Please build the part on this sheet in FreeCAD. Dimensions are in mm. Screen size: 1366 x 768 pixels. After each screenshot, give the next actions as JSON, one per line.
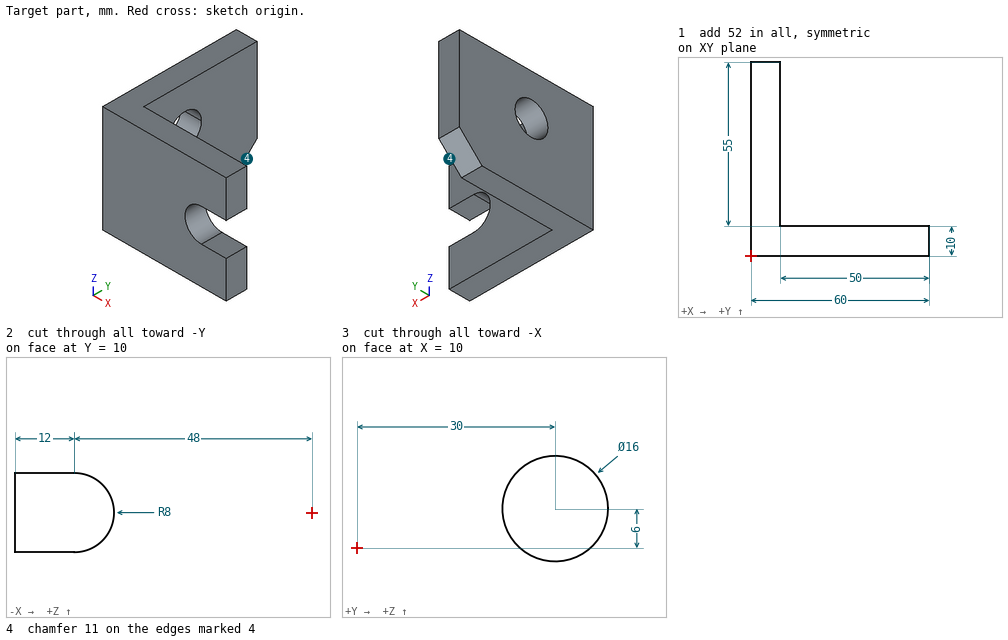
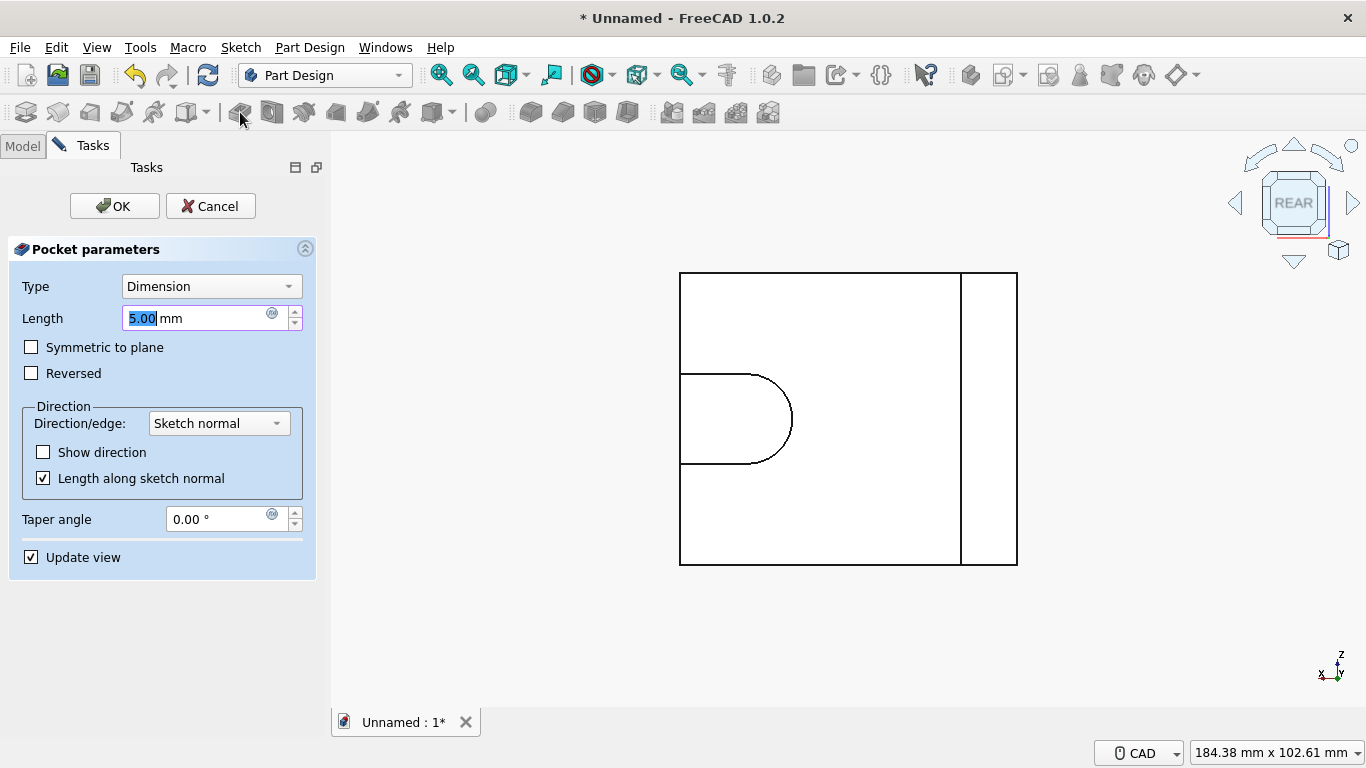
{"action": "left_click", "coordinate": [212, 286]}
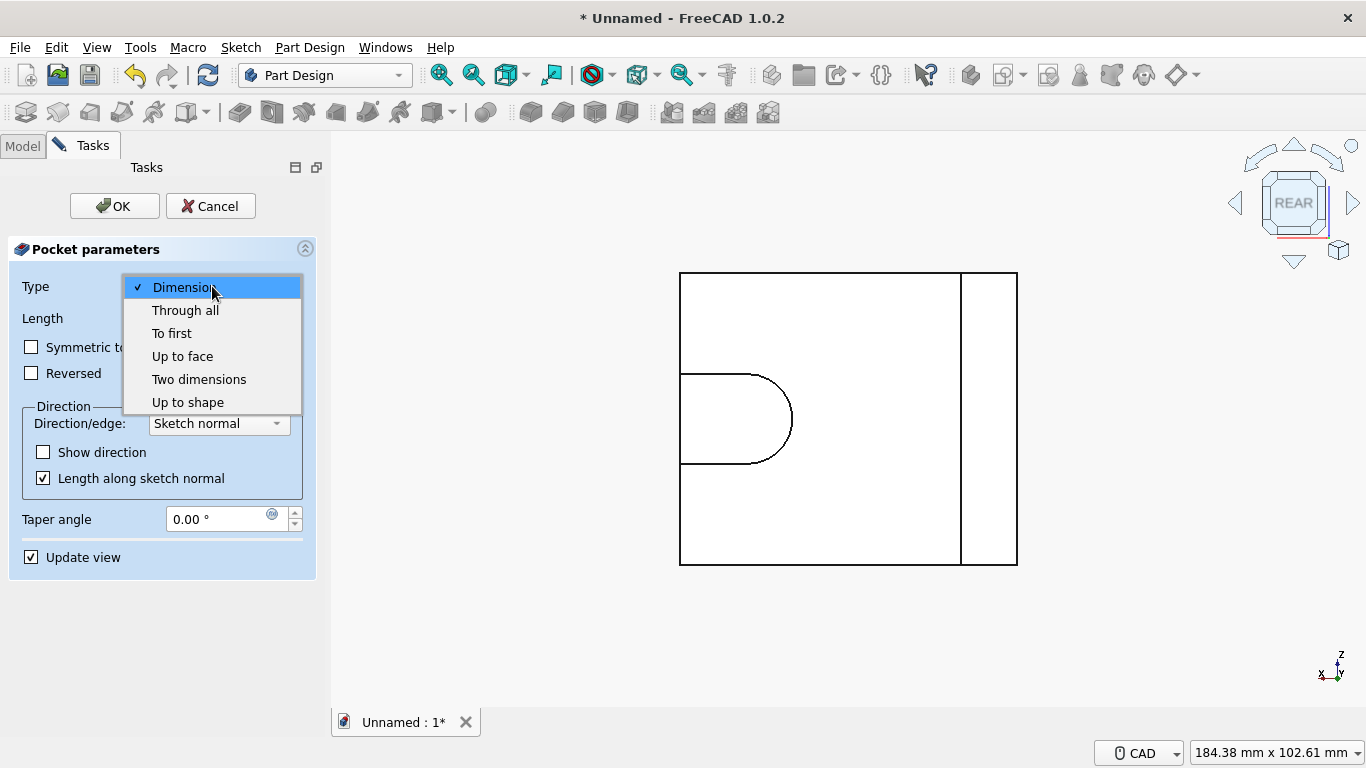
{"action": "left_click", "coordinate": [212, 310]}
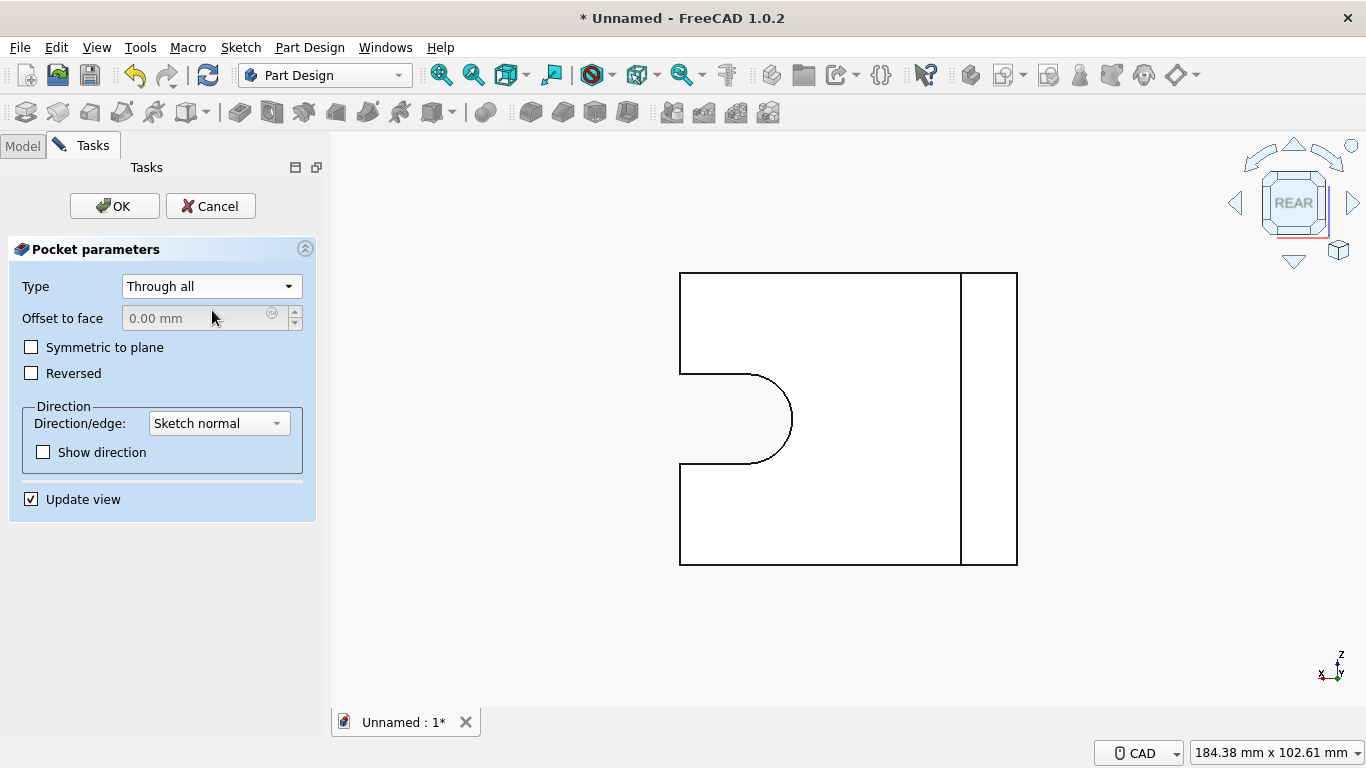
{"action": "left_click", "coordinate": [115, 206]}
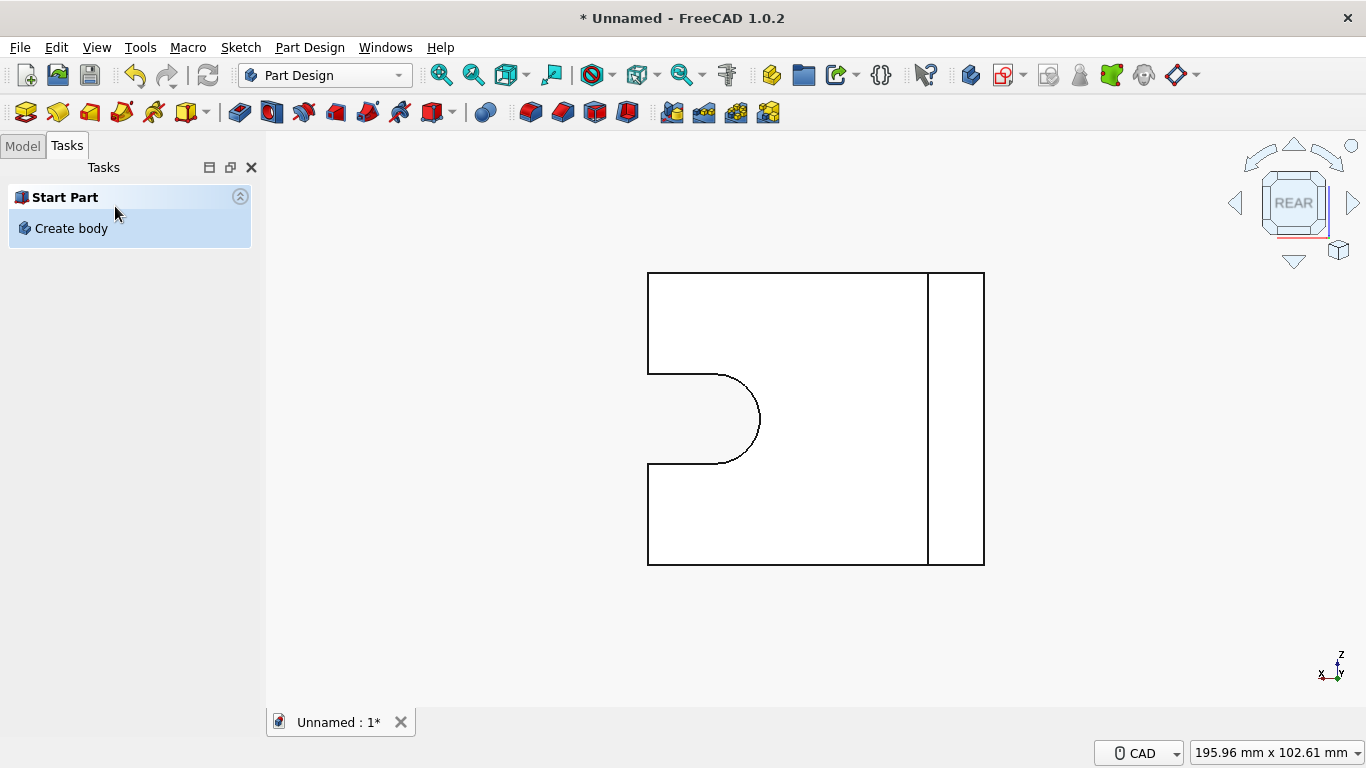
{"action": "key", "text": "0"}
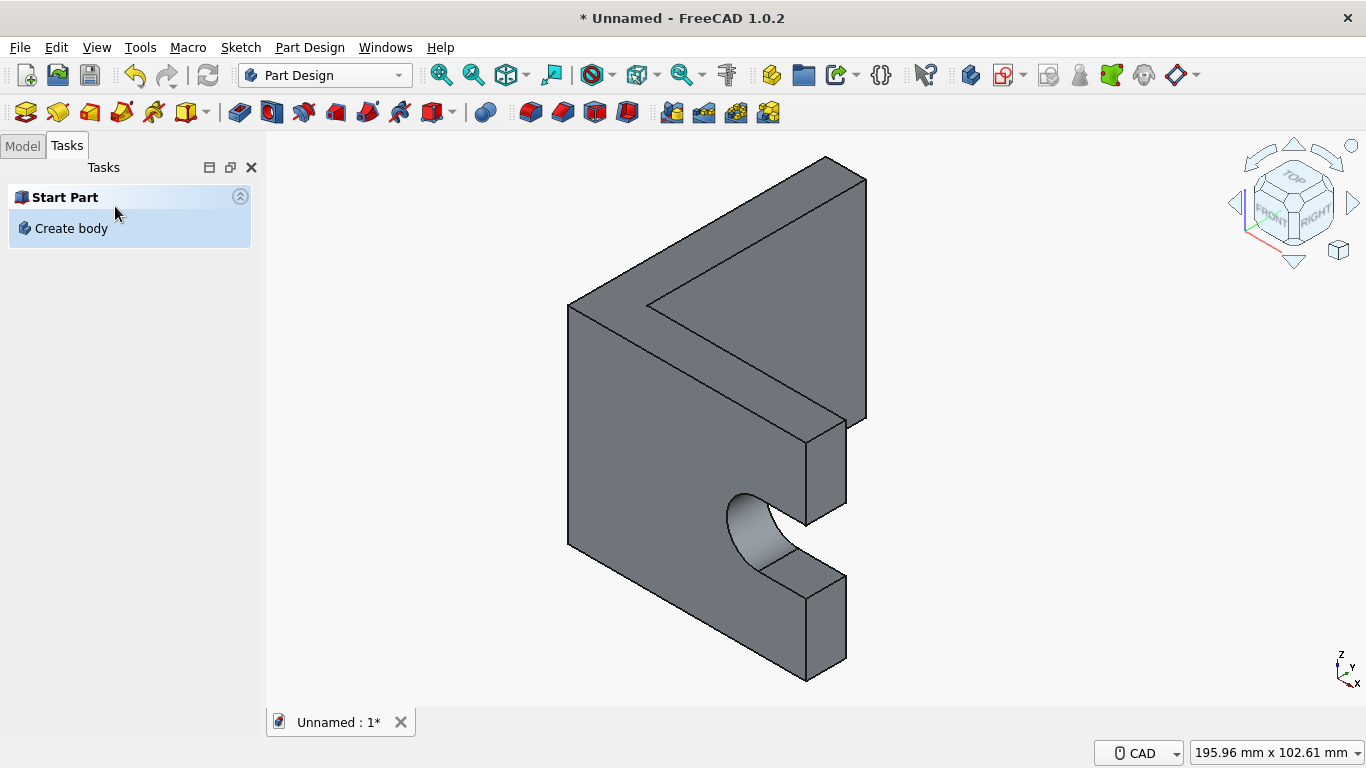
{"action": "left_click", "coordinate": [788, 343]}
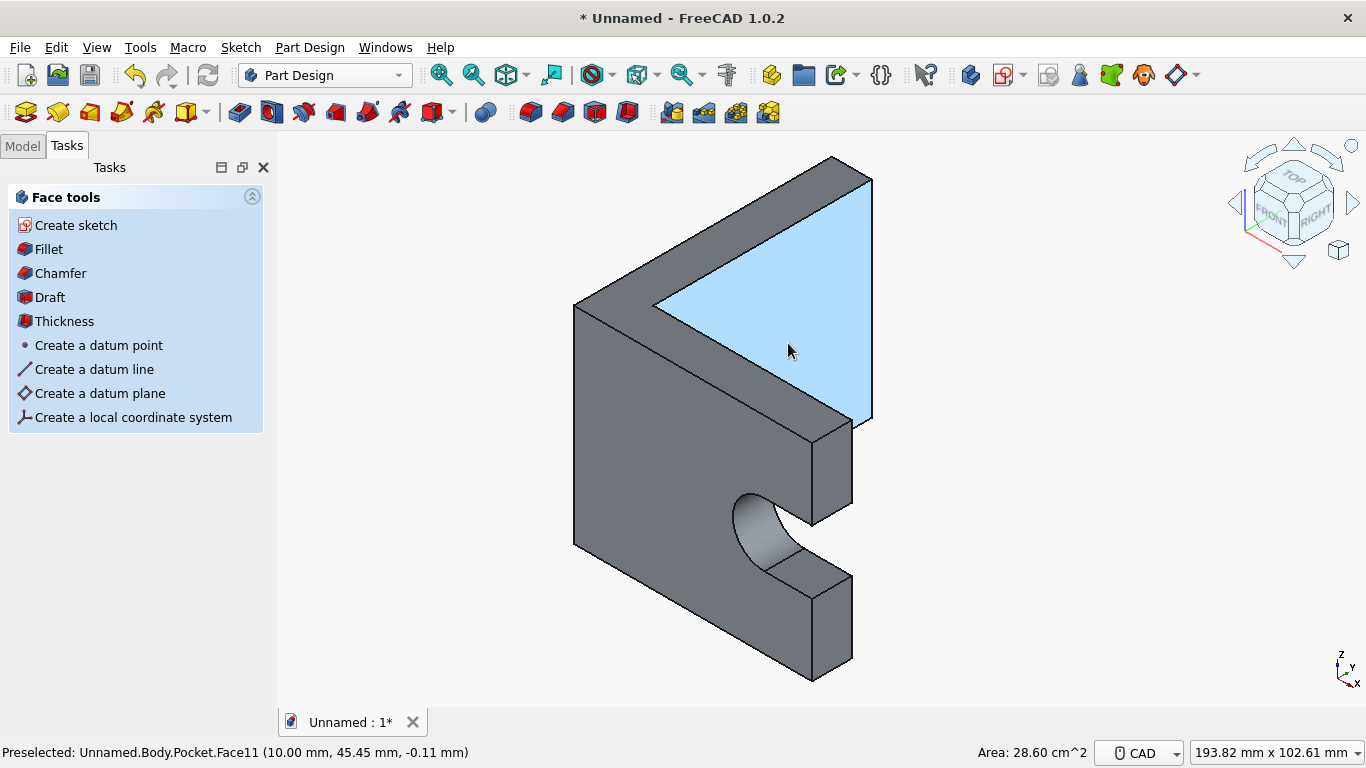
{"action": "left_click", "coordinate": [1004, 76]}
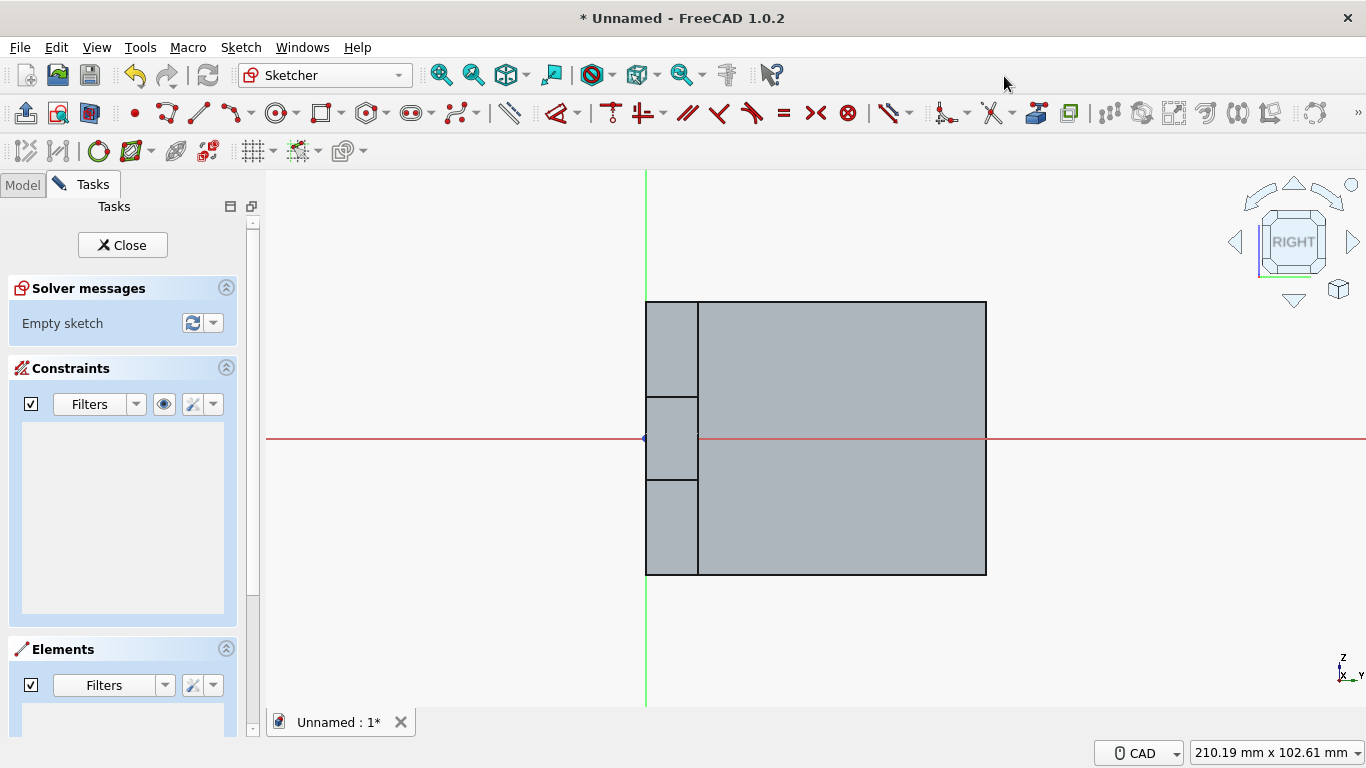
{"action": "scroll", "coordinate": [744, 394], "scroll_direction": "up", "scroll_amount": 6}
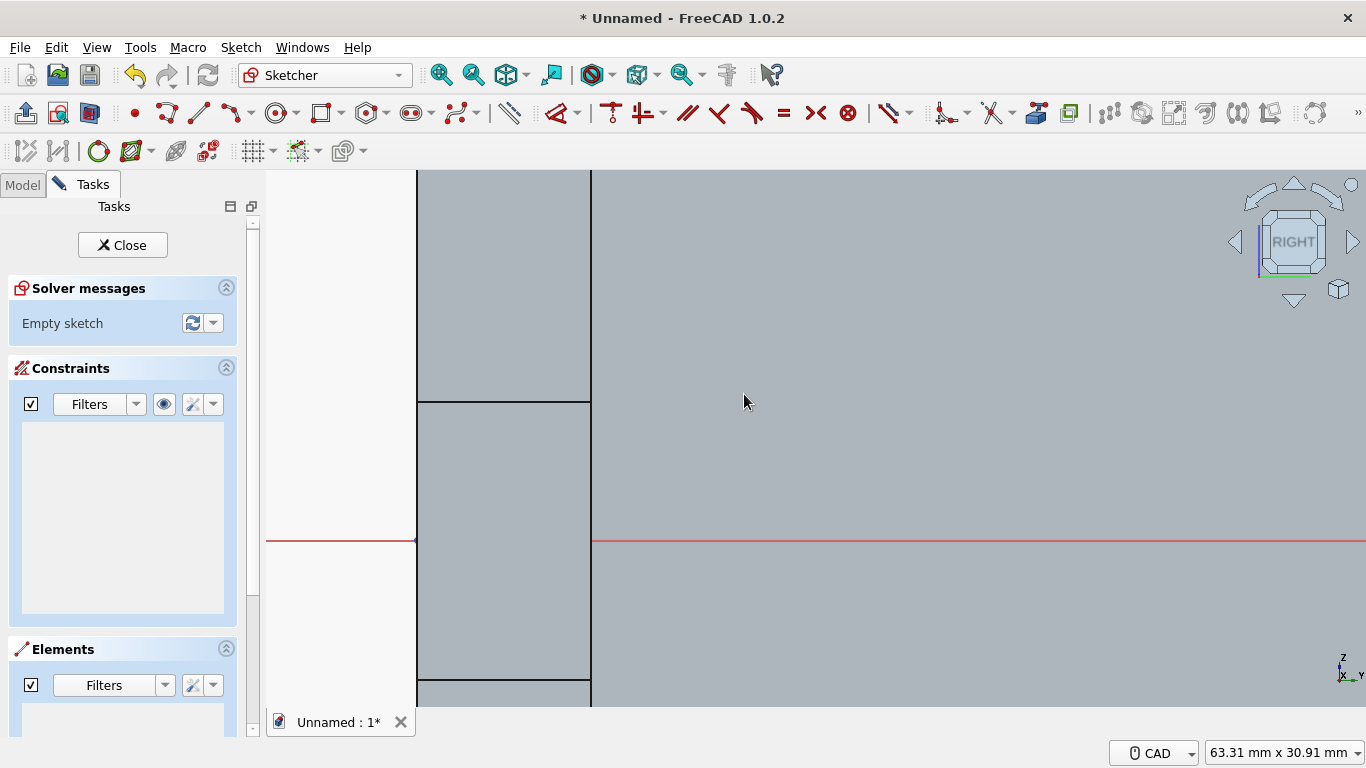
{"action": "left_click", "coordinate": [276, 114]}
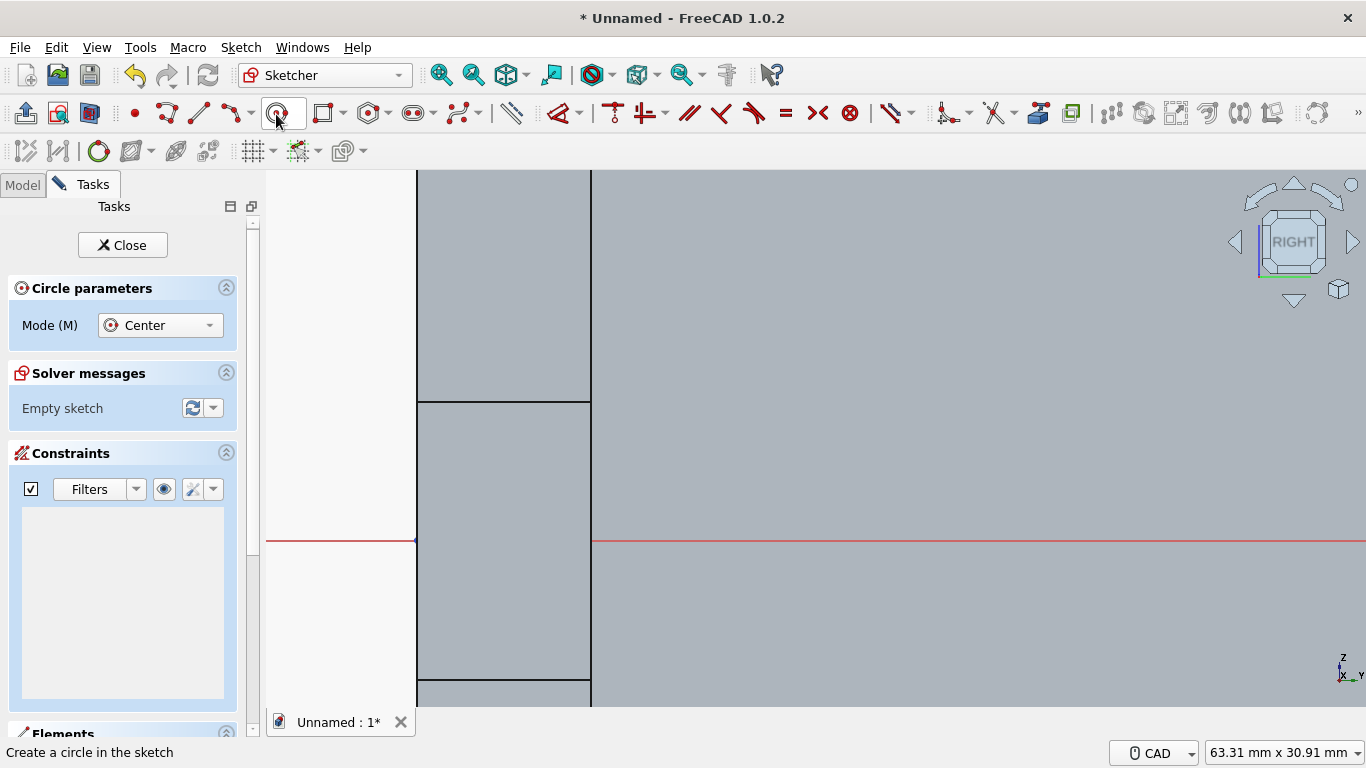
{"action": "left_click", "coordinate": [939, 437]}
{"action": "left_click", "coordinate": [1037, 338]}
{"action": "key", "text": "Escape"}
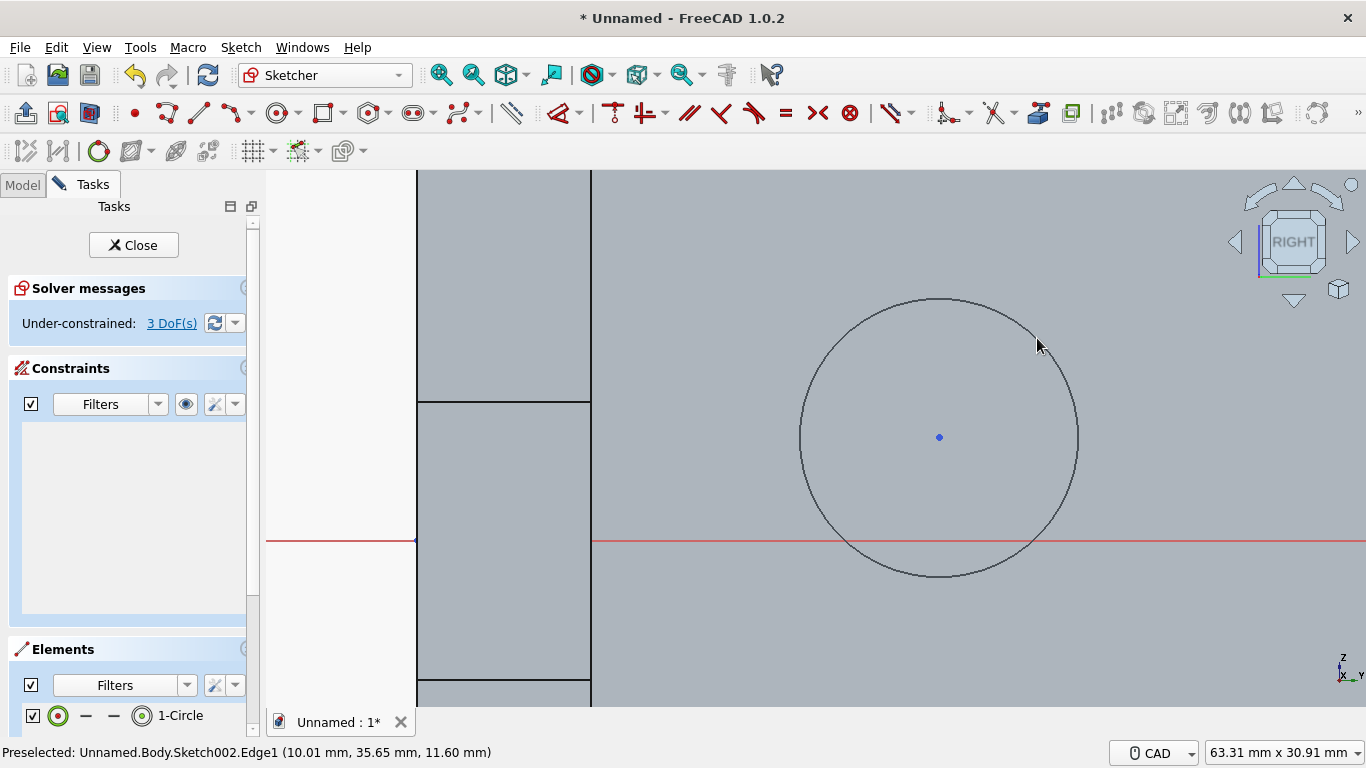
{"action": "left_click", "coordinate": [558, 114]}